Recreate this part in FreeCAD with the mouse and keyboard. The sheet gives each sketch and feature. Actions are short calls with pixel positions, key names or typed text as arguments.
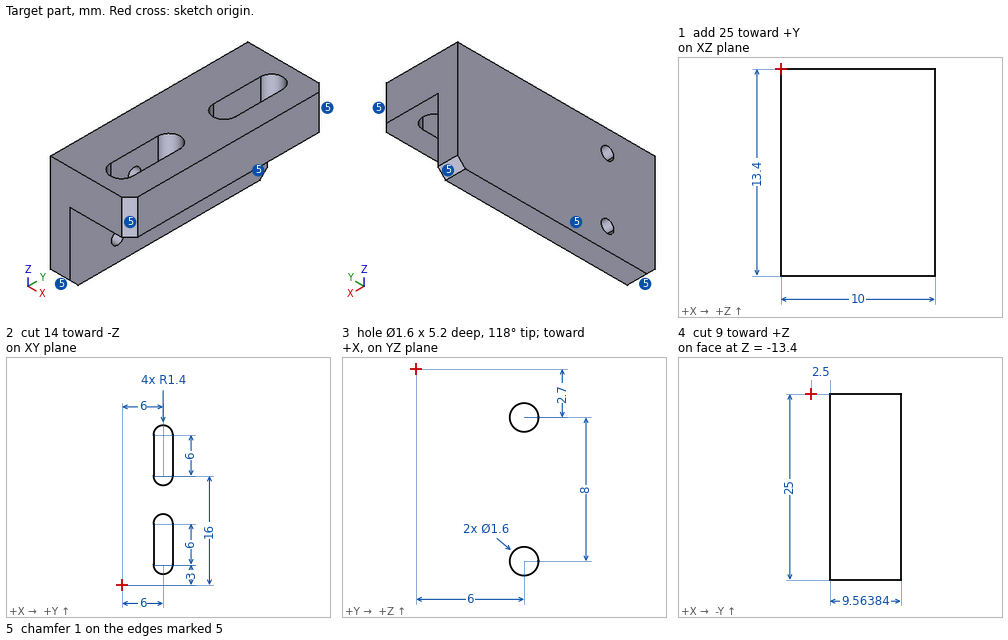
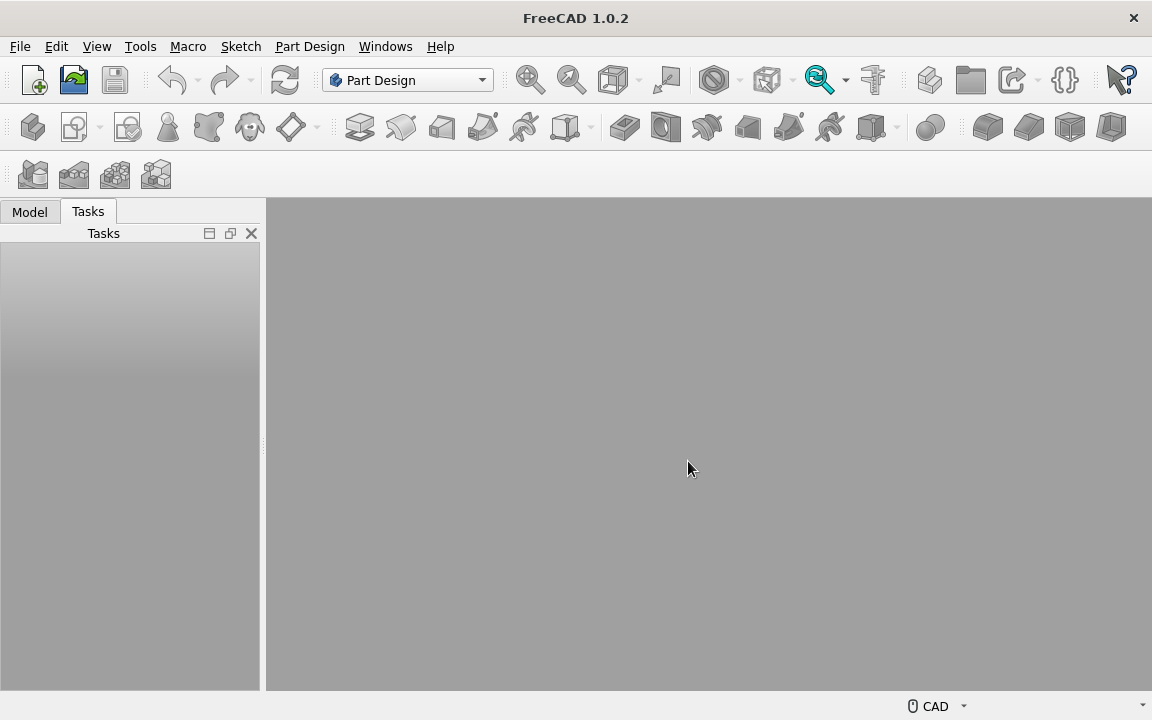
click(33, 80)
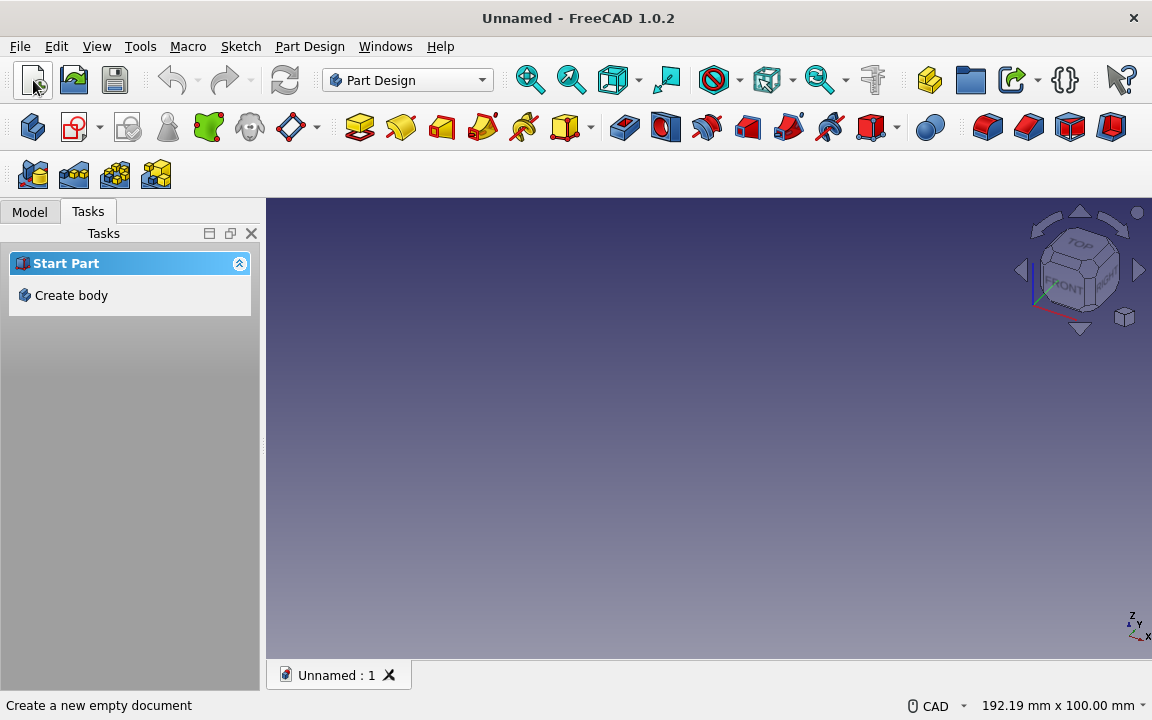
click(74, 128)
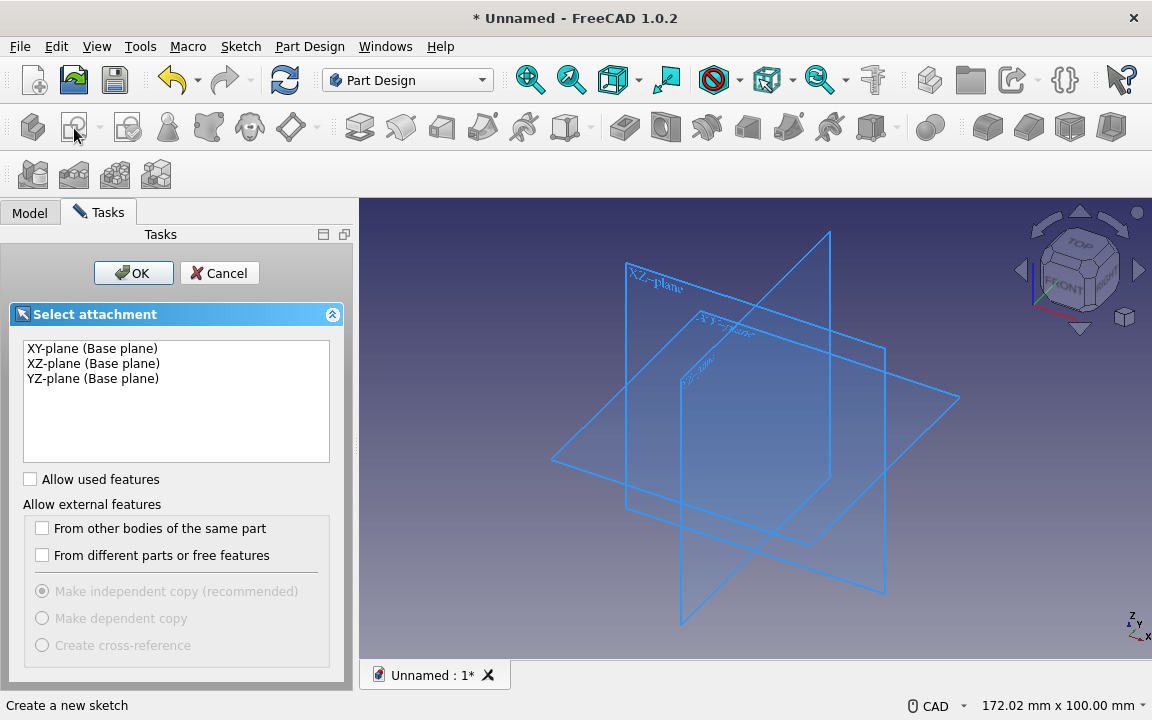
click(84, 364)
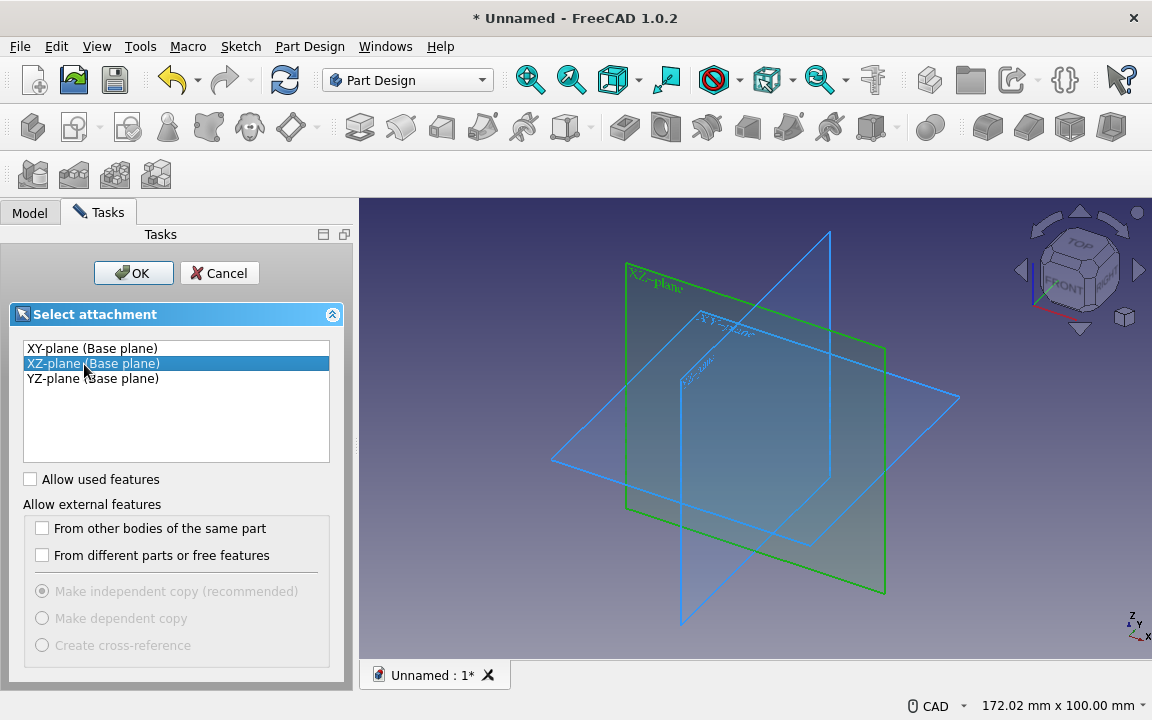
click(134, 273)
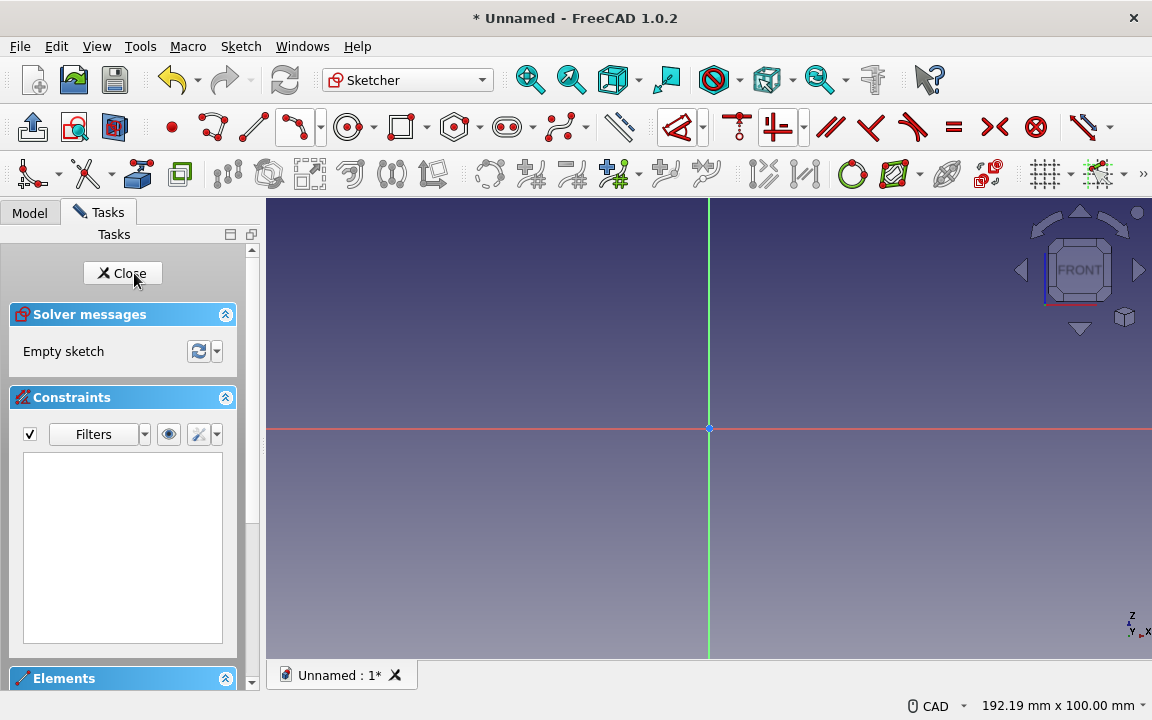
scroll(755, 467, up, 8)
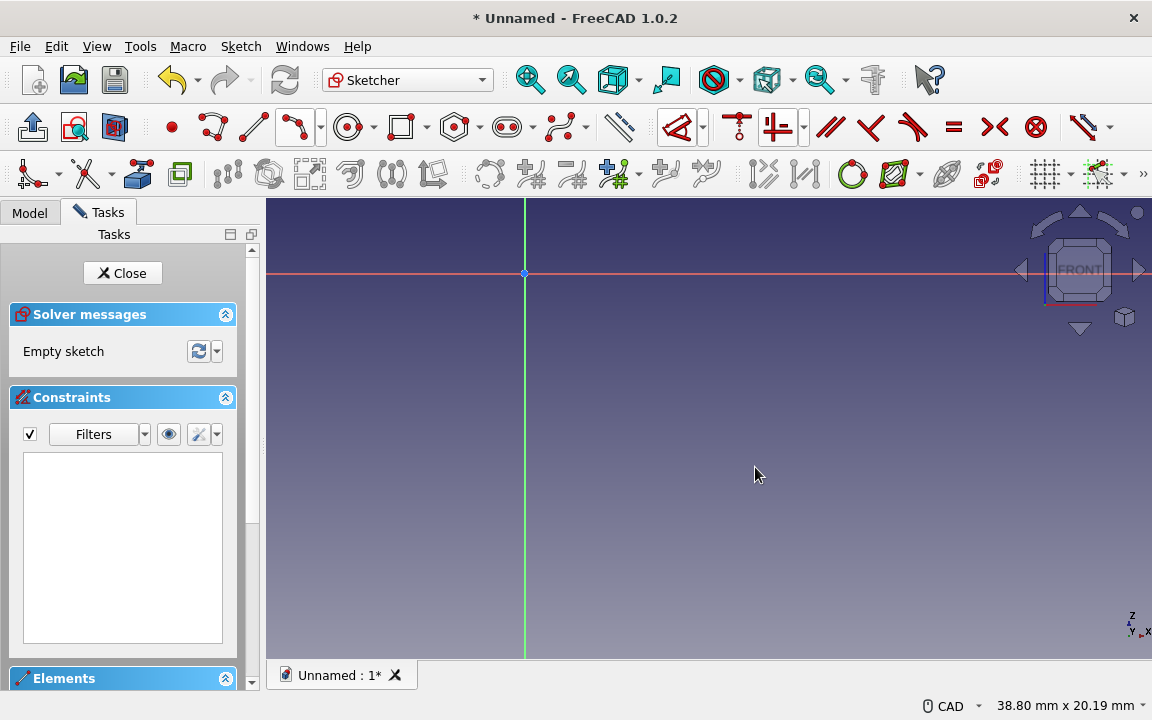
click(400, 128)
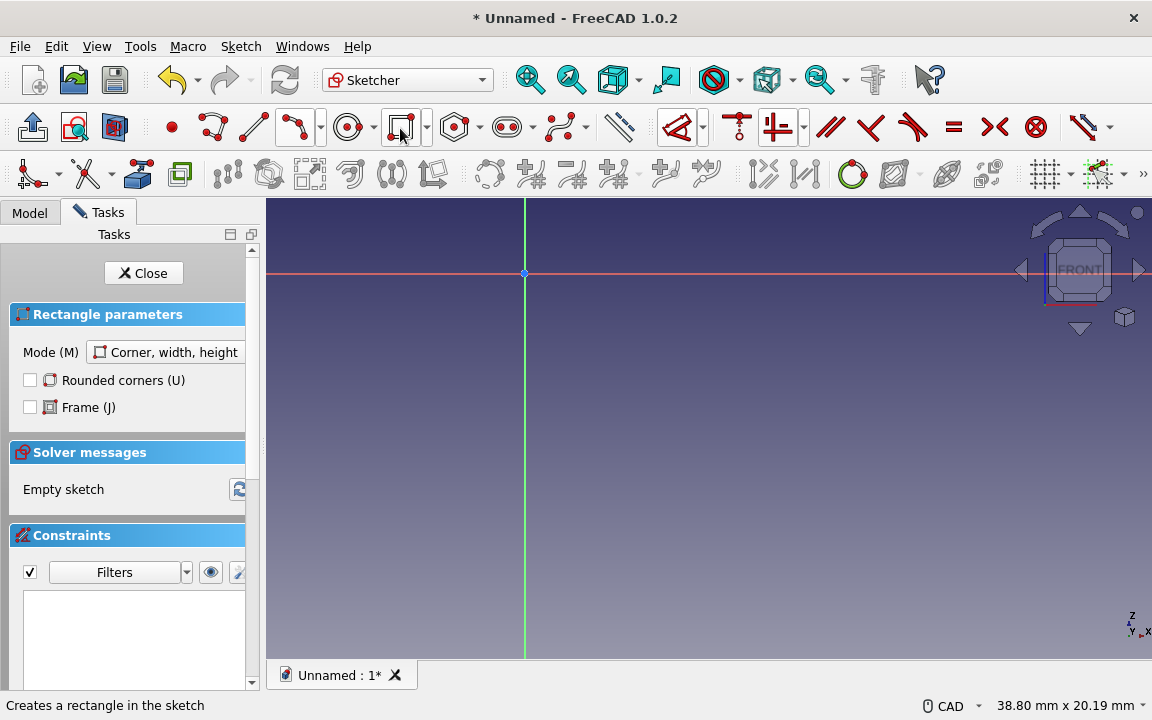
click(525, 274)
click(753, 580)
key(Escape)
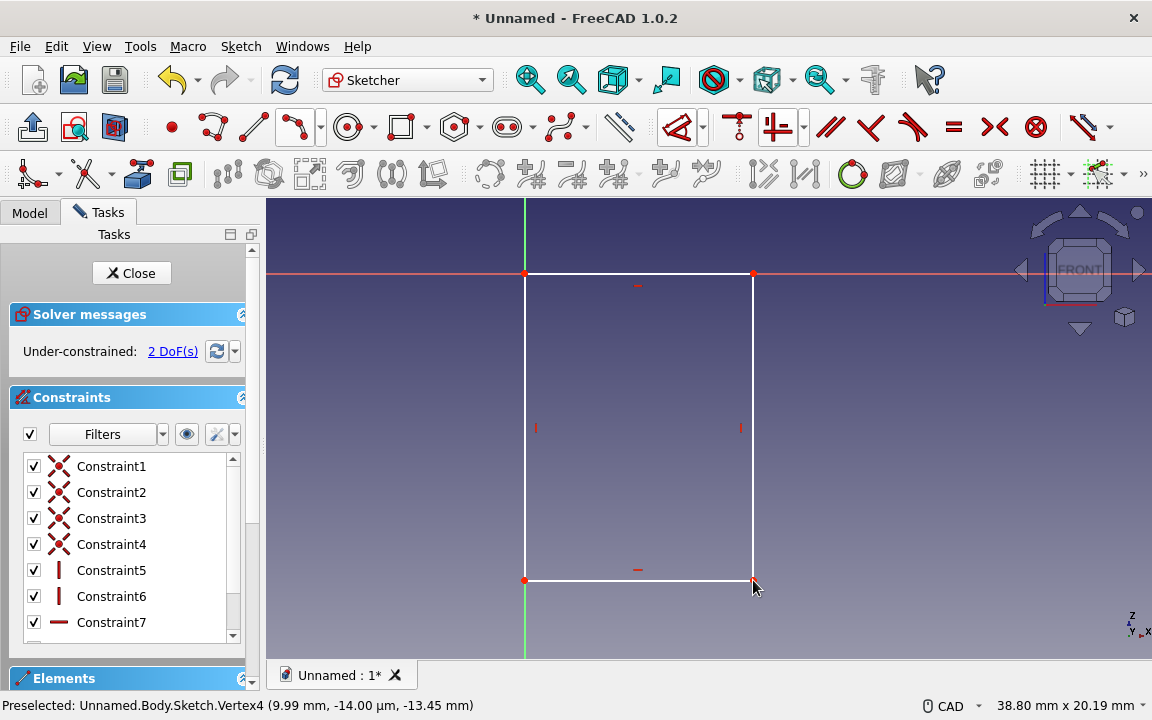
click(676, 128)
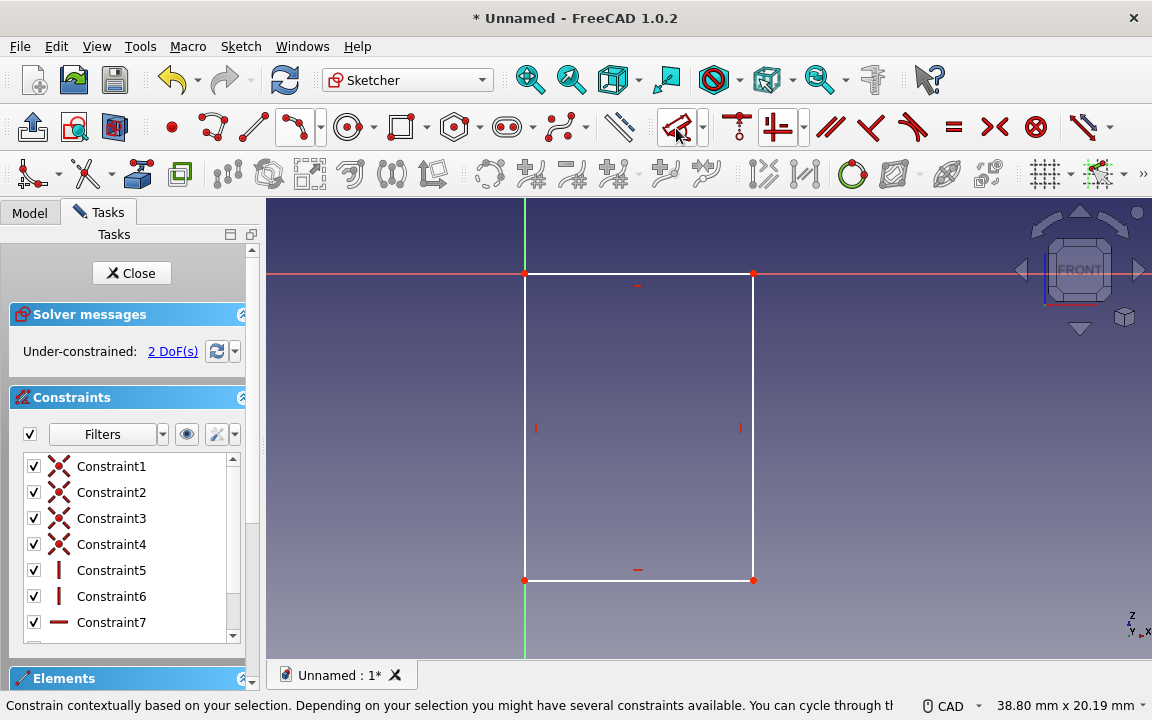
click(593, 581)
click(639, 615)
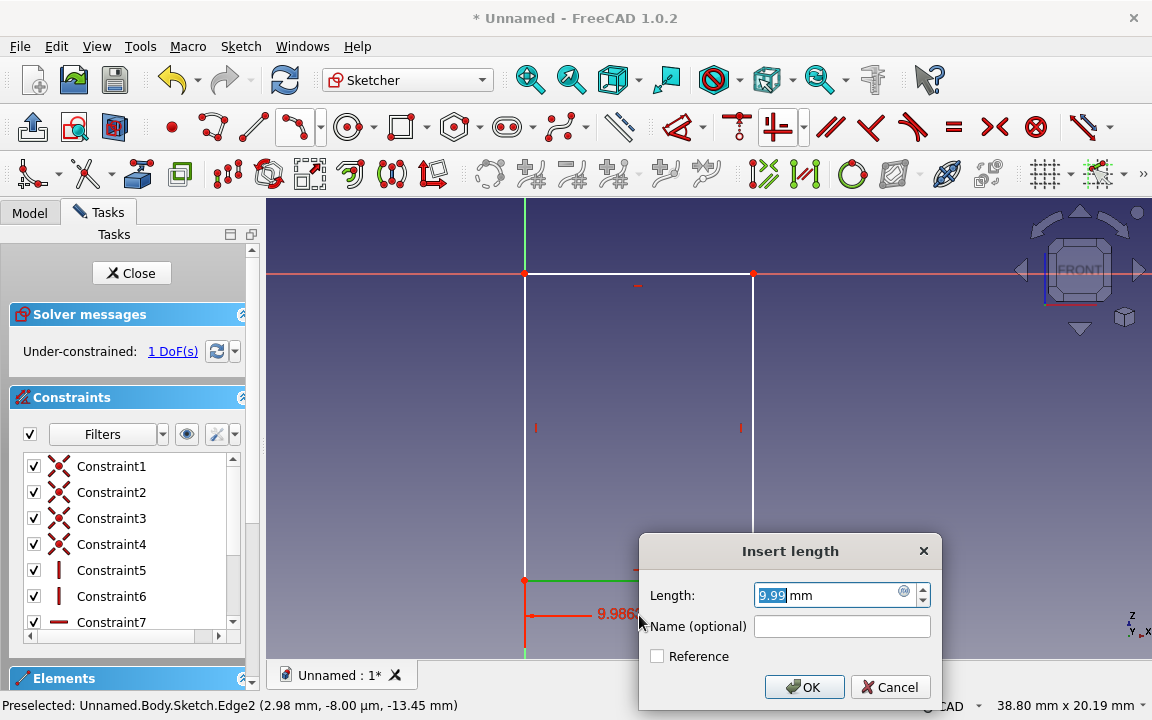
text(10)
key(Return)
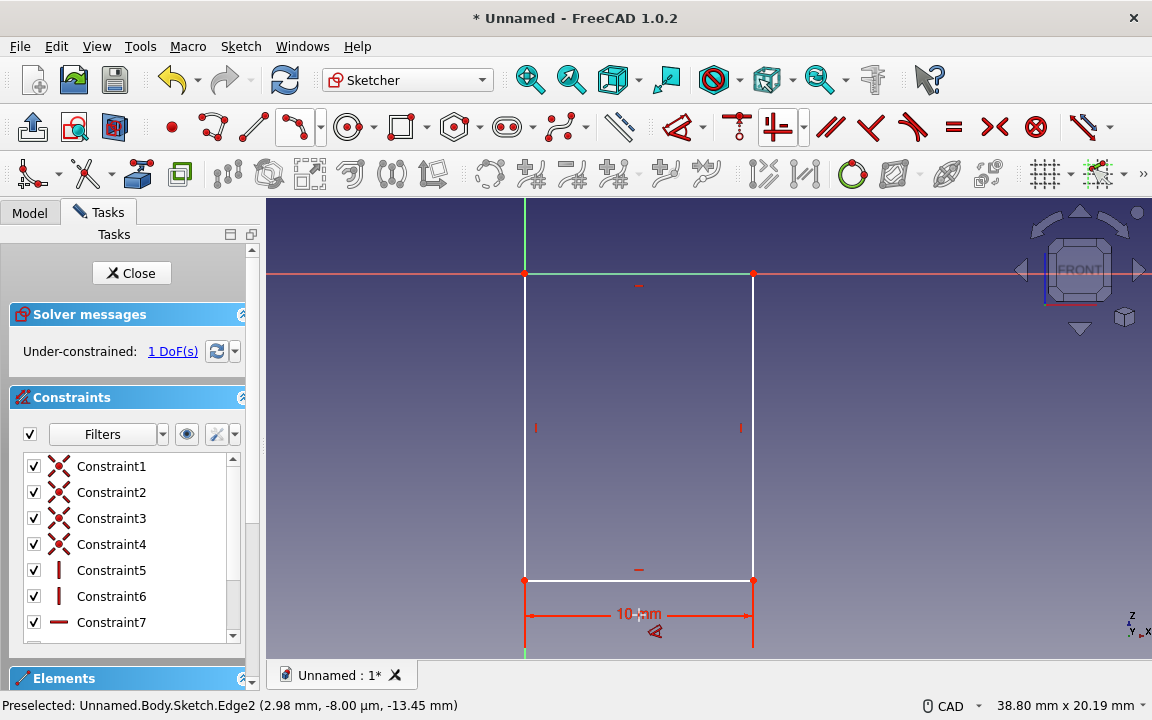
click(525, 366)
click(491, 427)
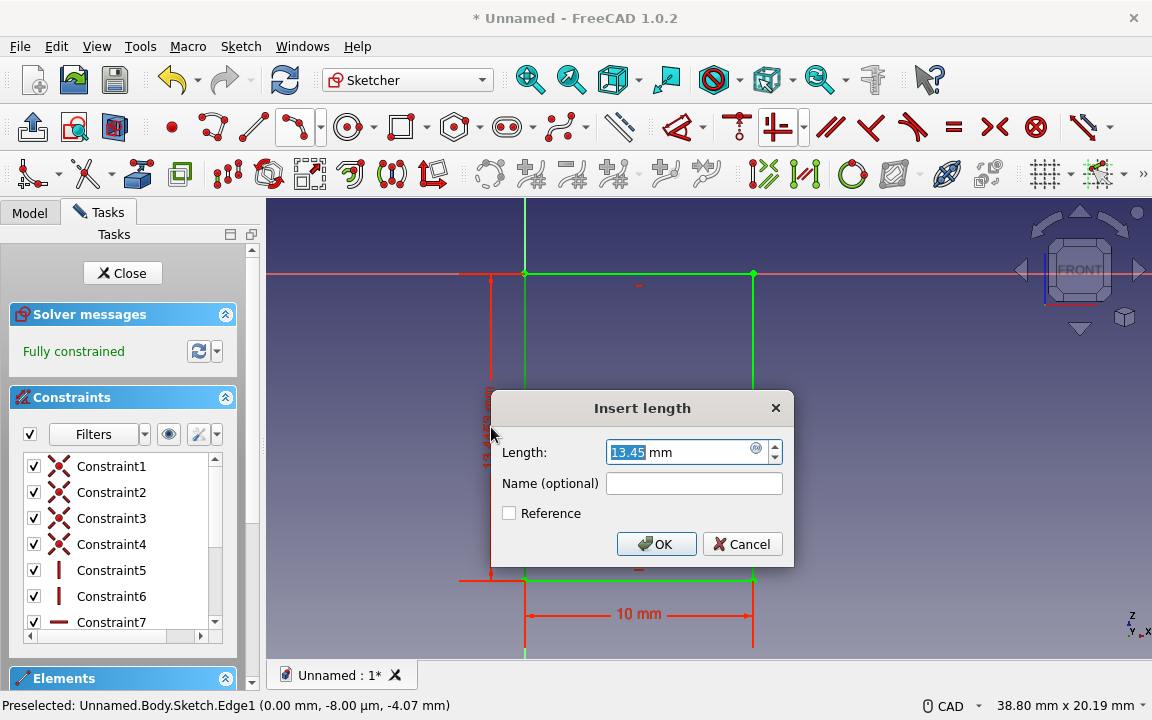
text(13.4)
key(Return)
key(Escape)